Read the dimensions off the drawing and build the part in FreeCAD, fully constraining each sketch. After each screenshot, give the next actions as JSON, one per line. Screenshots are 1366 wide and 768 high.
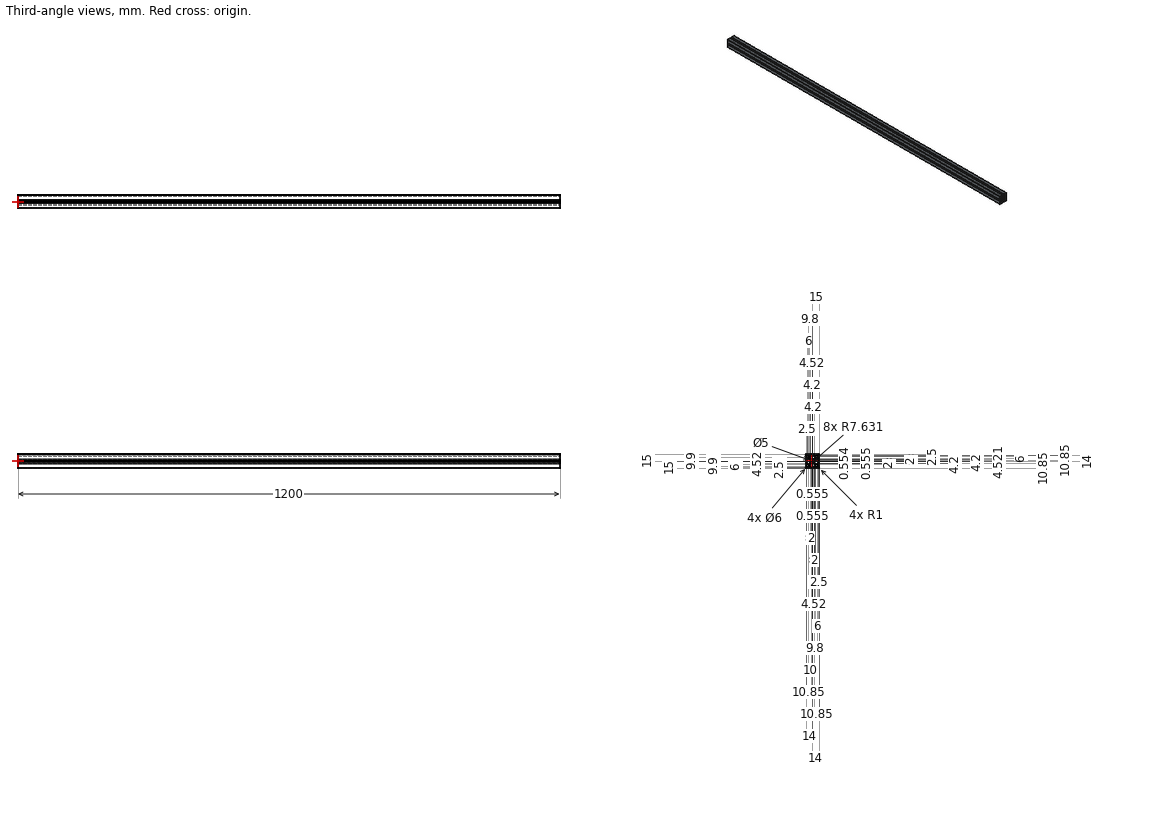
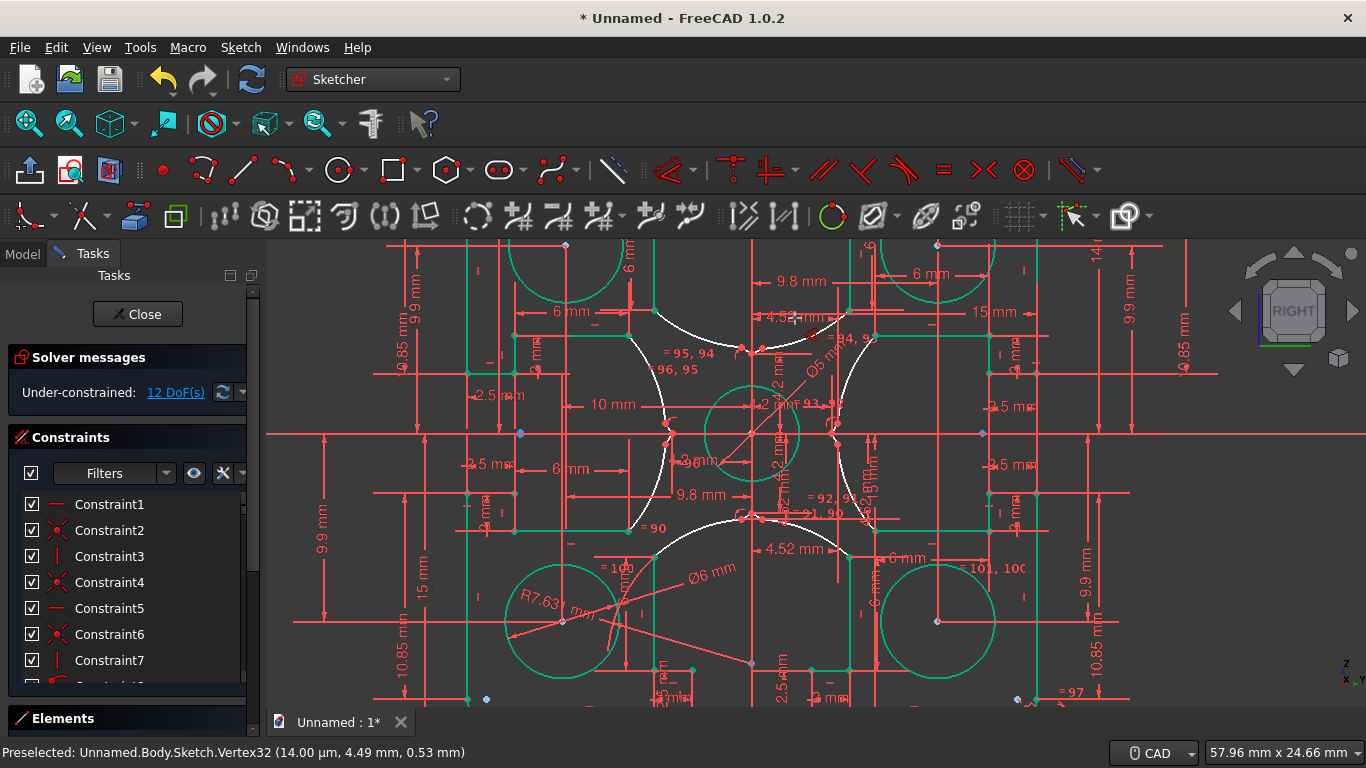
{"action": "left_click", "coordinate": [665, 424]}
{"action": "left_click", "coordinate": [689, 390]}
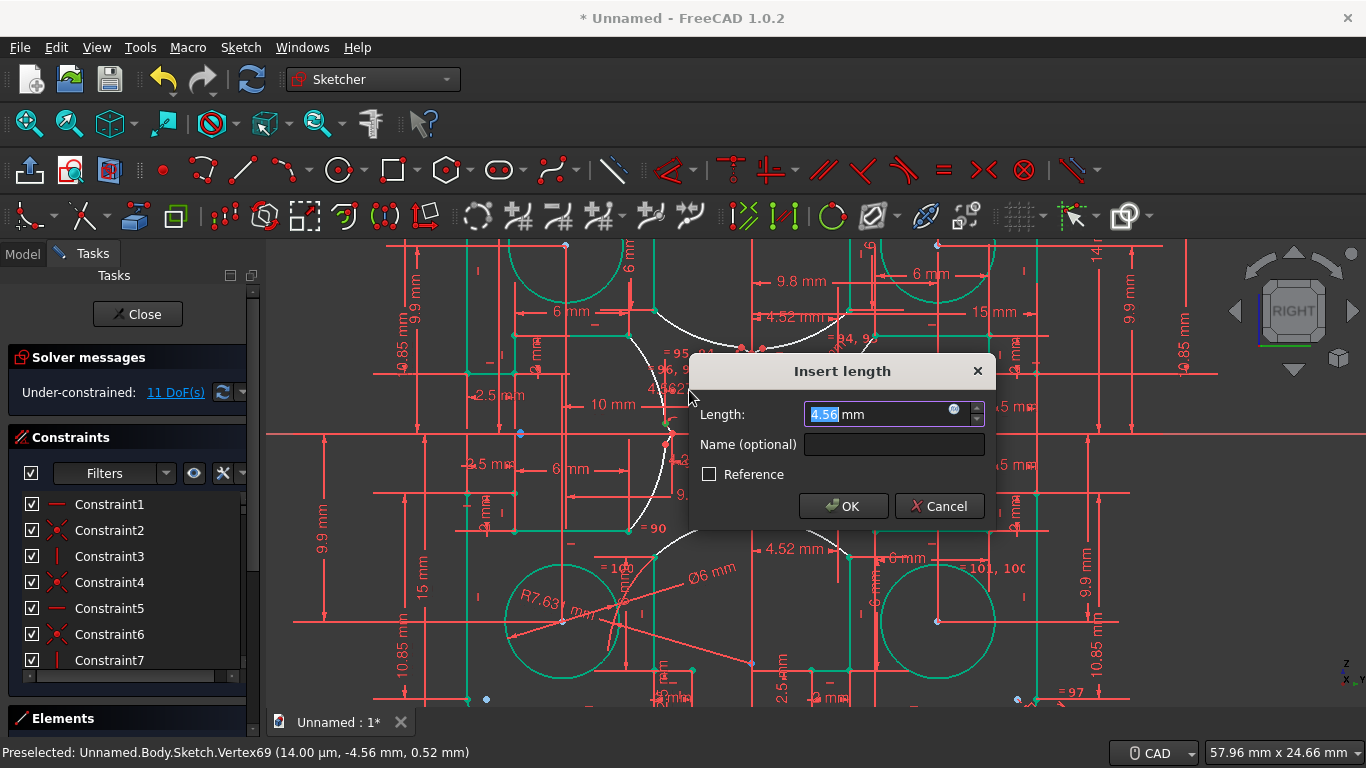
{"action": "type", "text": "4.52"}
{"action": "key", "text": "Return"}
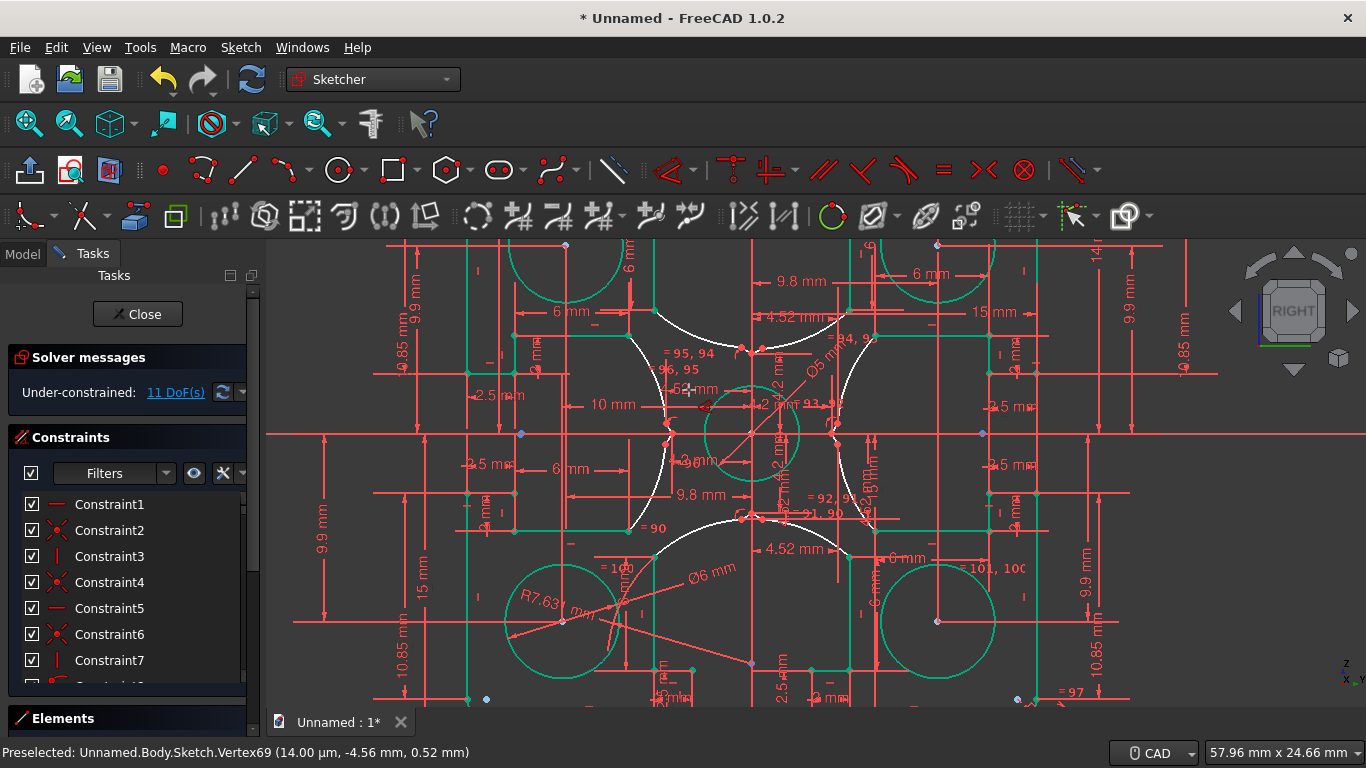
{"action": "left_click", "coordinate": [665, 445]}
{"action": "left_click", "coordinate": [689, 352]}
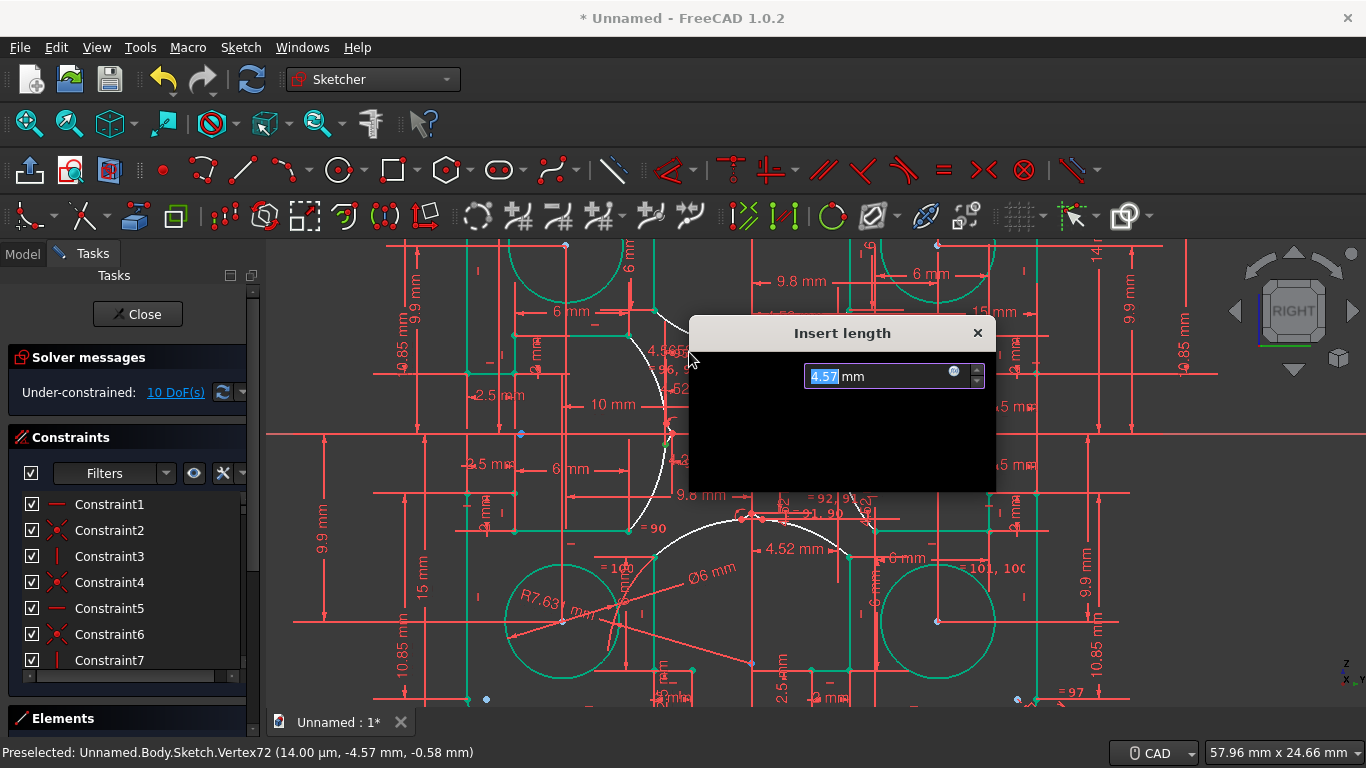
{"action": "type", "text": "4.52"}
{"action": "key", "text": "Return"}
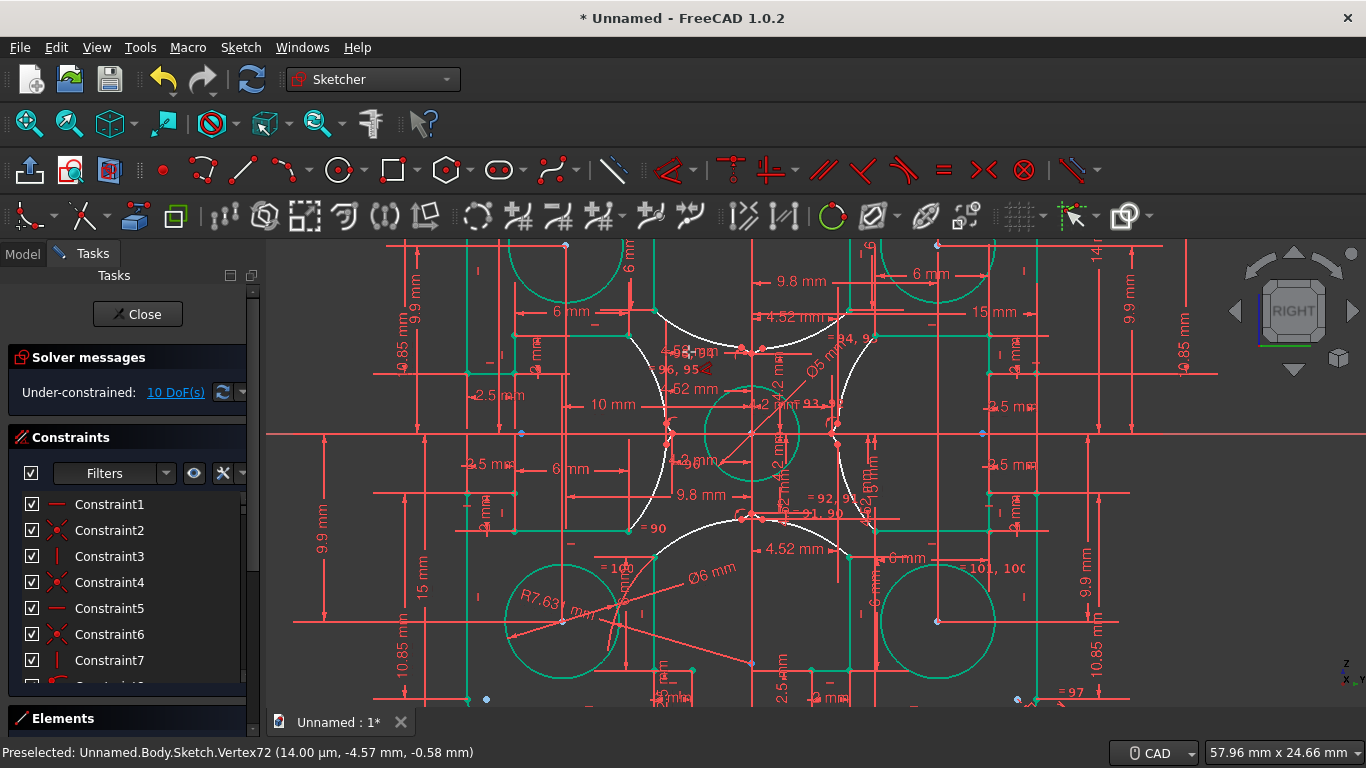
{"action": "scroll", "coordinate": [741, 519], "scroll_direction": "up", "scroll_amount": 7}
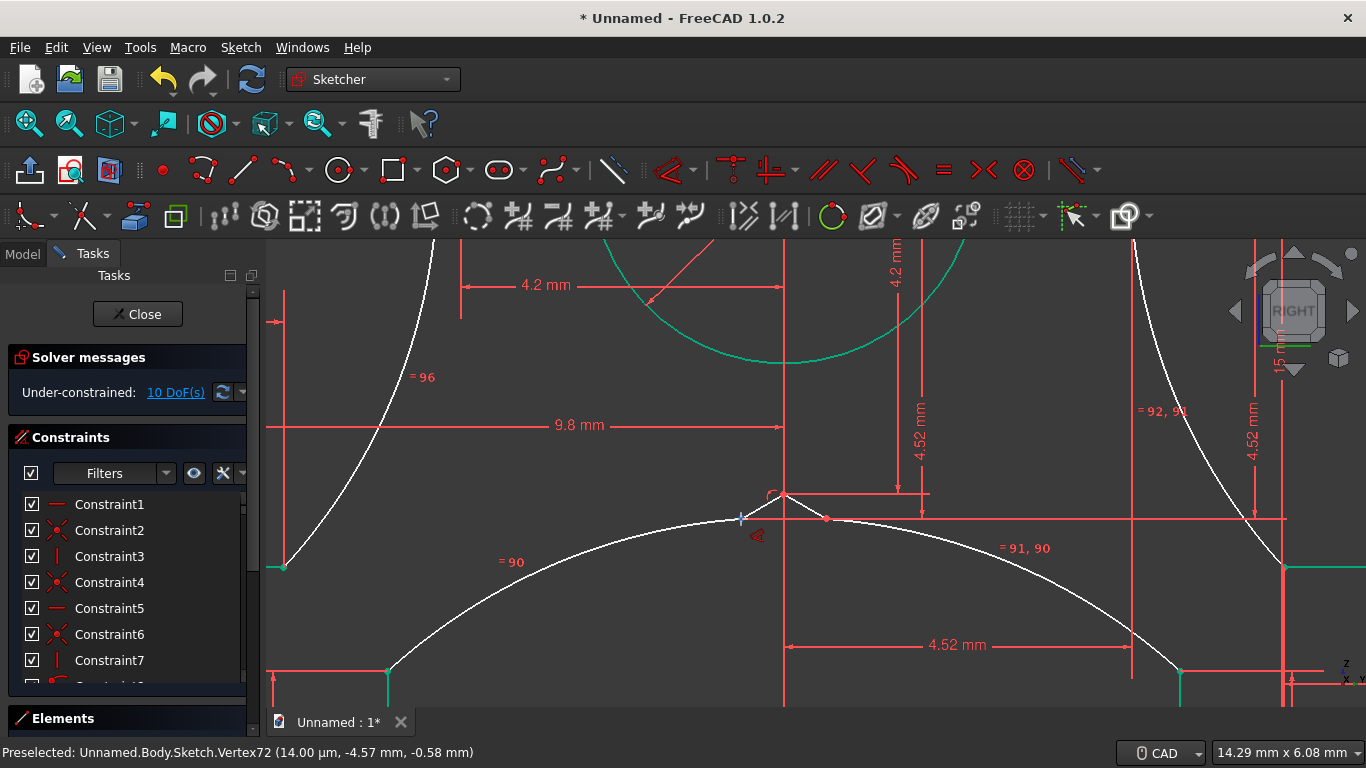
{"action": "left_click", "coordinate": [742, 519]}
{"action": "left_click", "coordinate": [763, 553]}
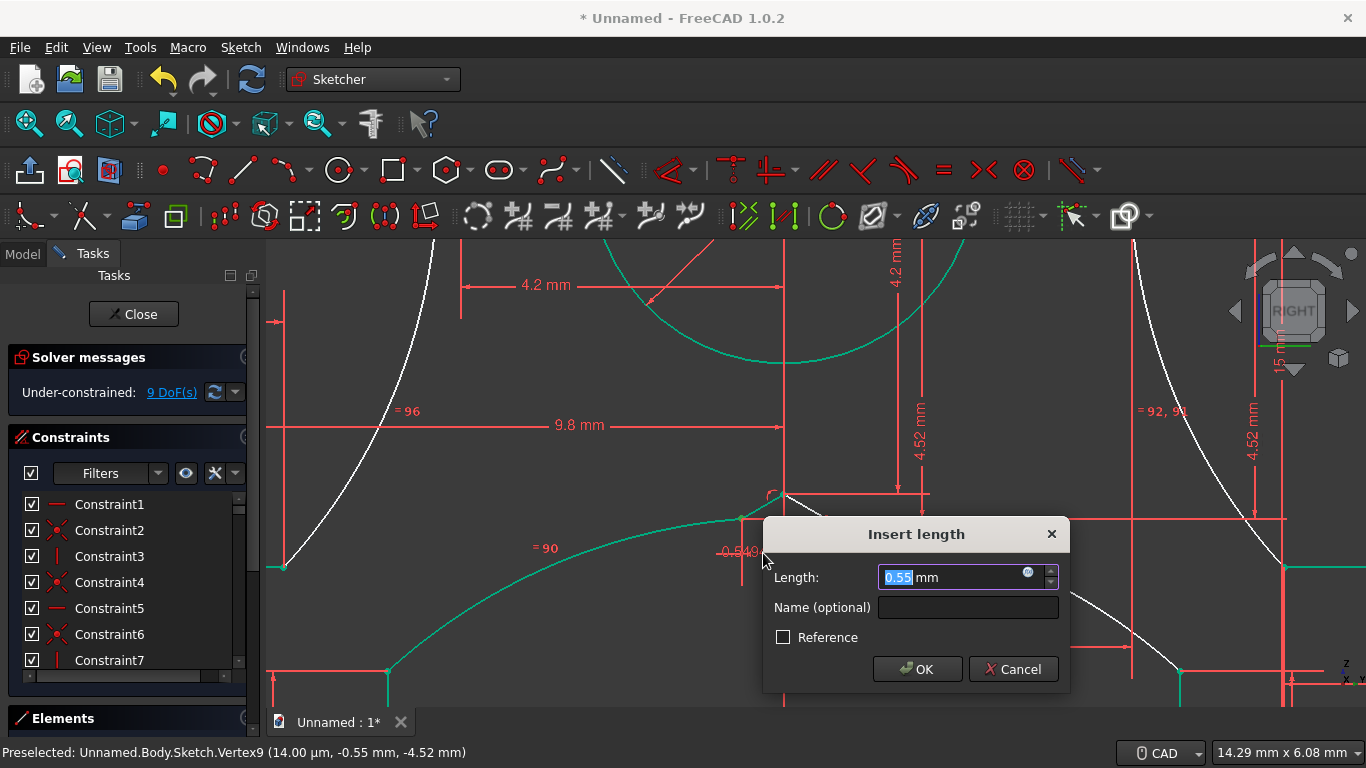
{"action": "type", "text": "0.555"}
{"action": "key", "text": "Return"}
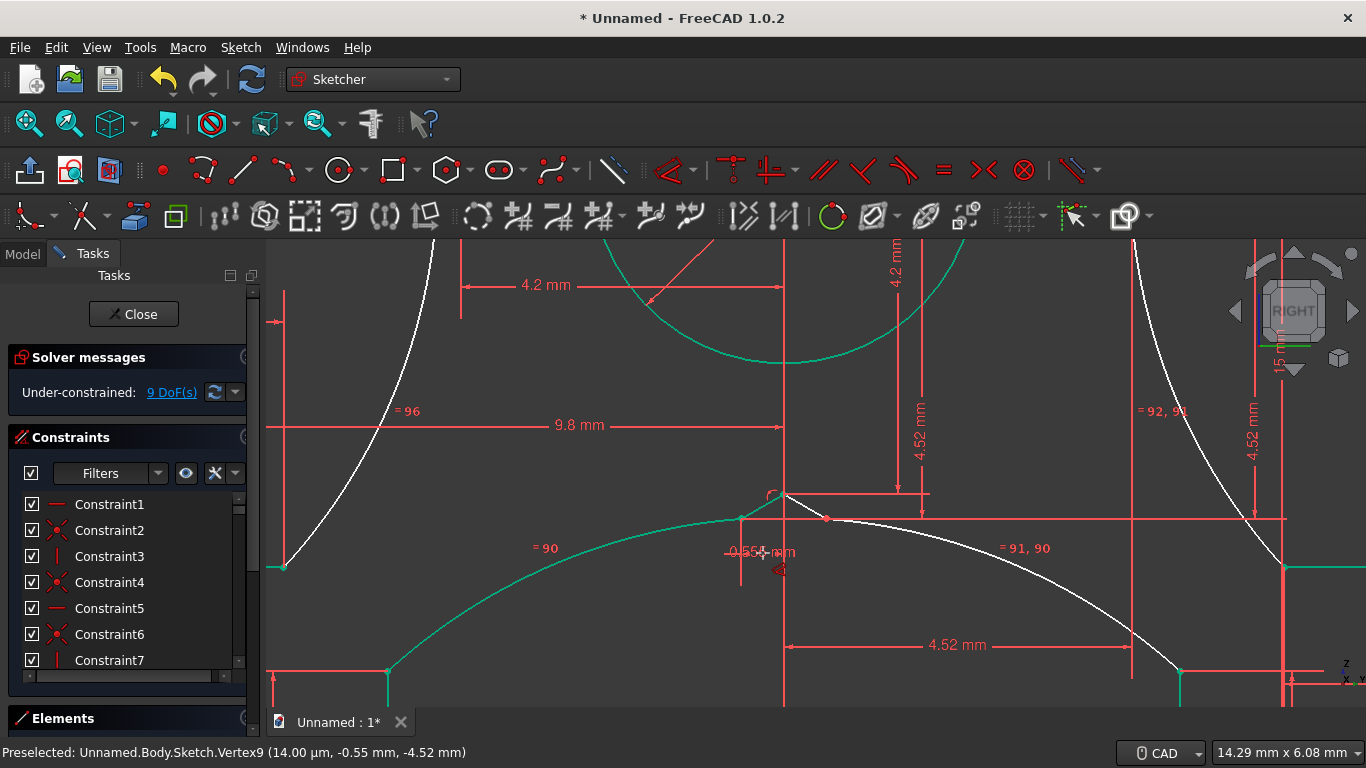
{"action": "left_click", "coordinate": [827, 519]}
{"action": "left_click", "coordinate": [805, 577]}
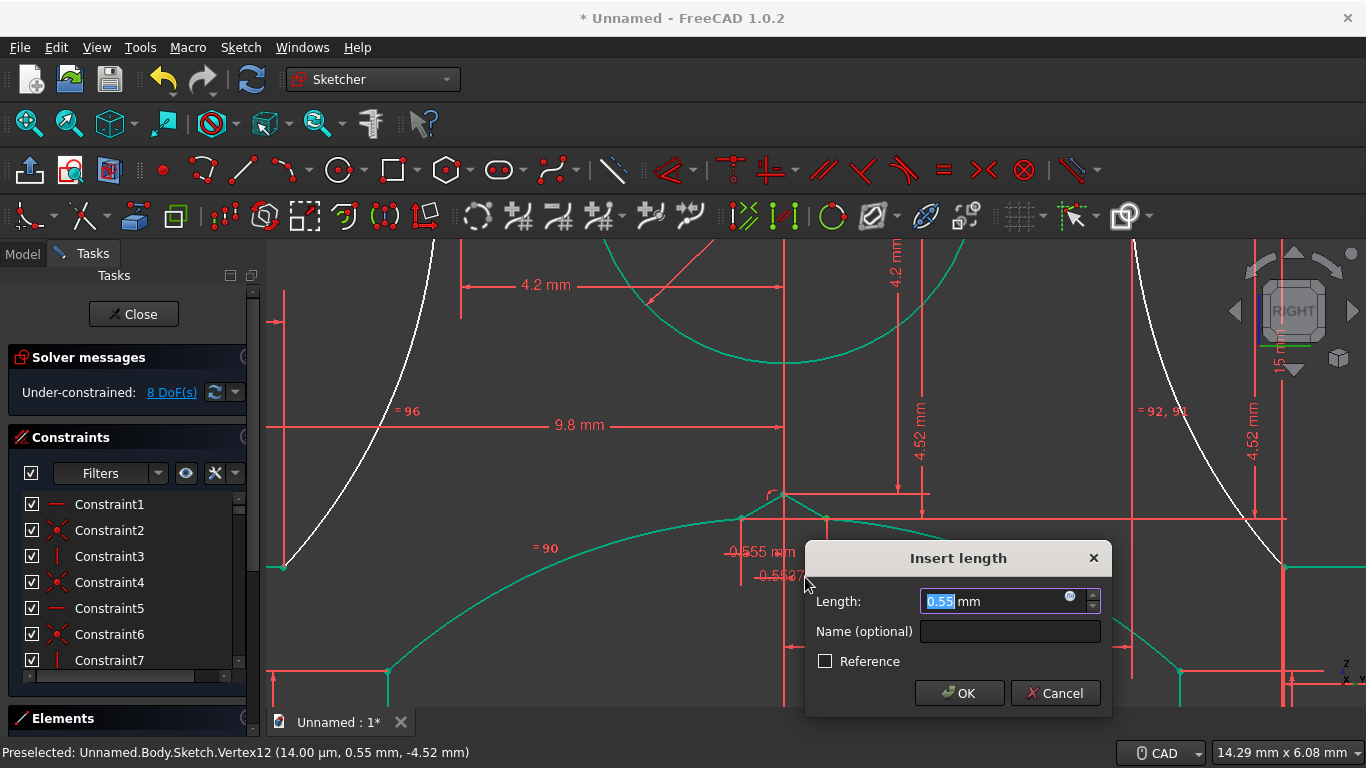
{"action": "type", "text": "0.555"}
{"action": "key", "text": "Return"}